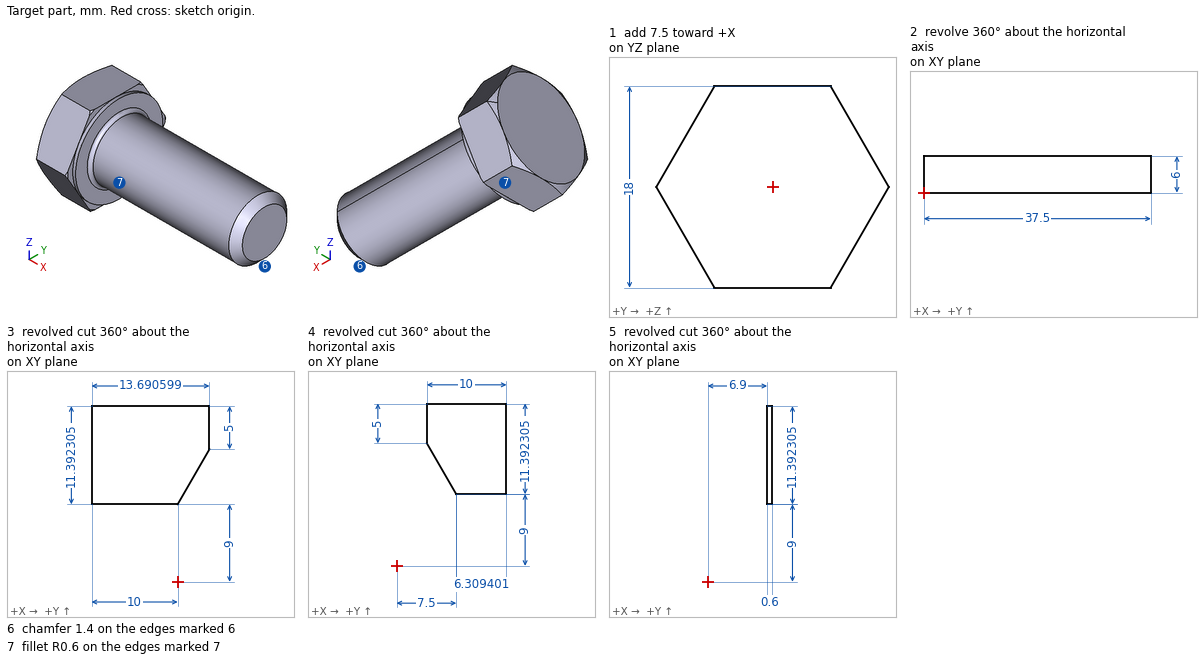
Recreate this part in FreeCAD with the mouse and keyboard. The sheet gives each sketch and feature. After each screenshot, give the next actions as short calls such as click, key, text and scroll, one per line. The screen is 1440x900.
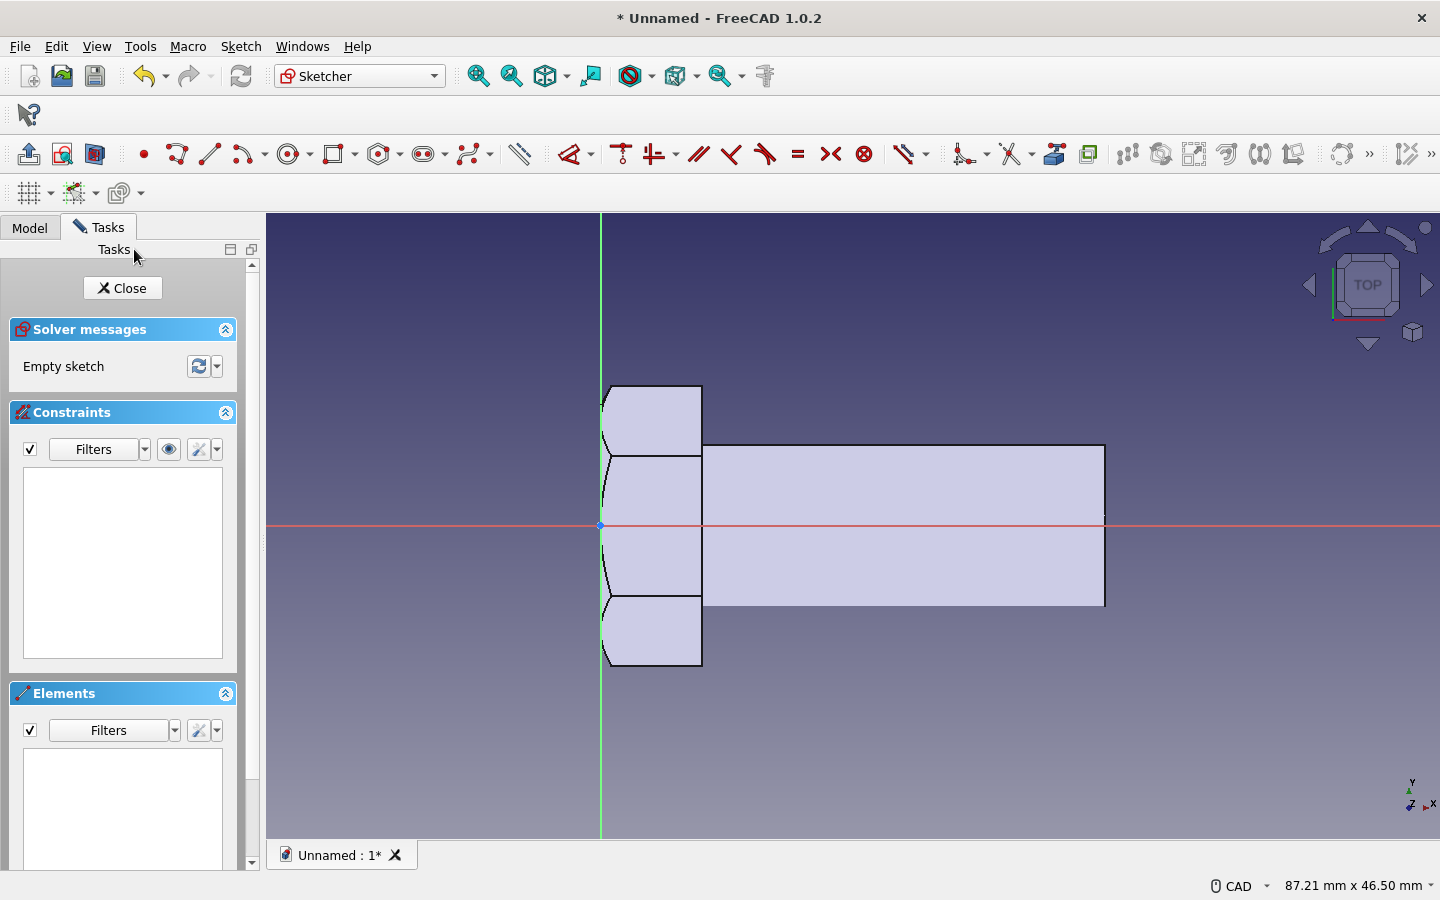
scroll(1195, 811, down, 1)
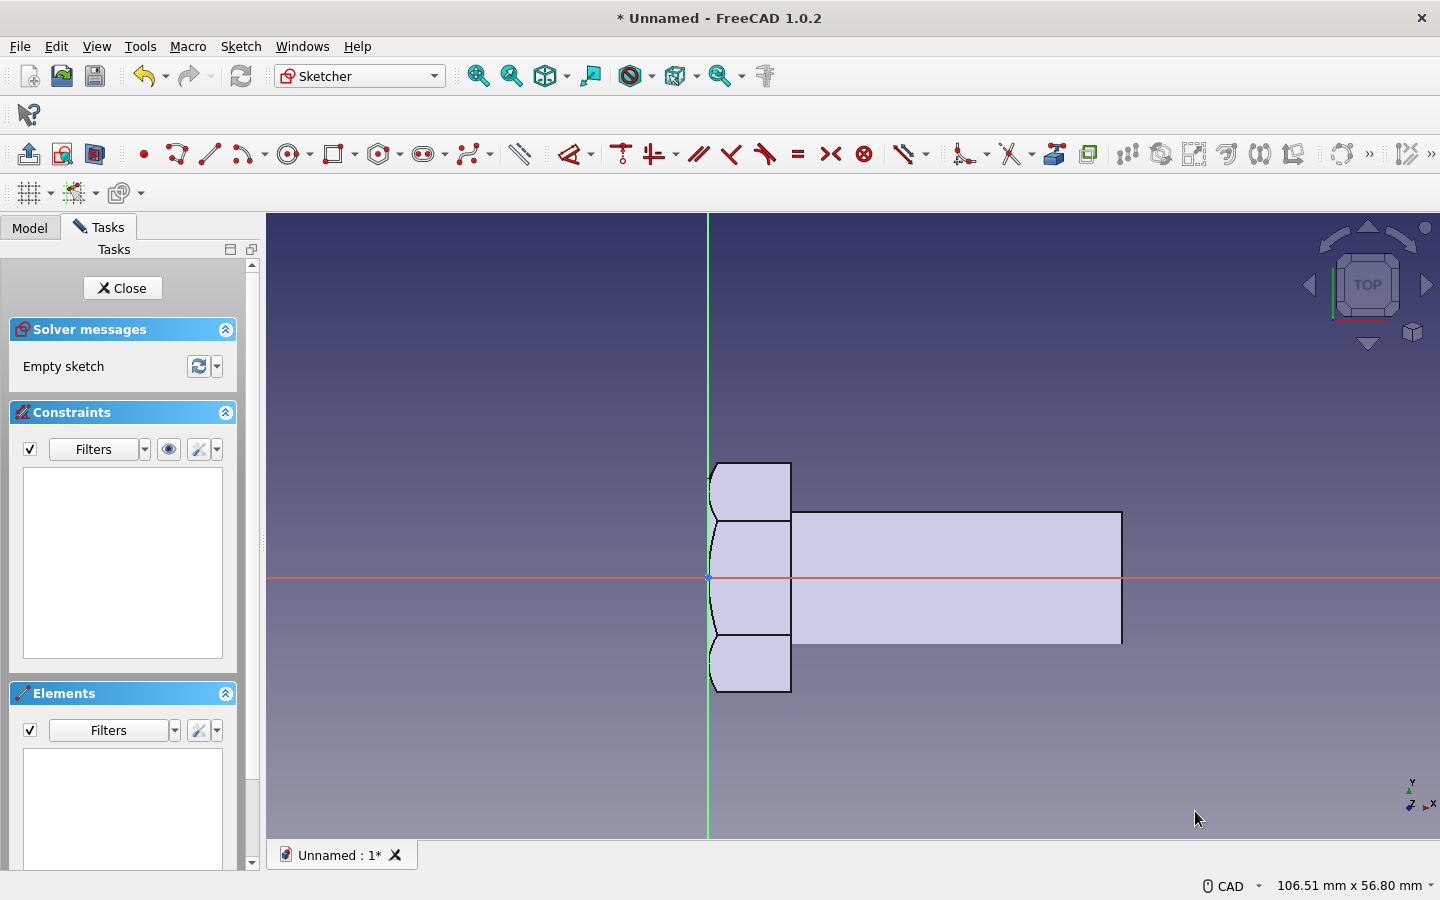
scroll(785, 392, up, 3)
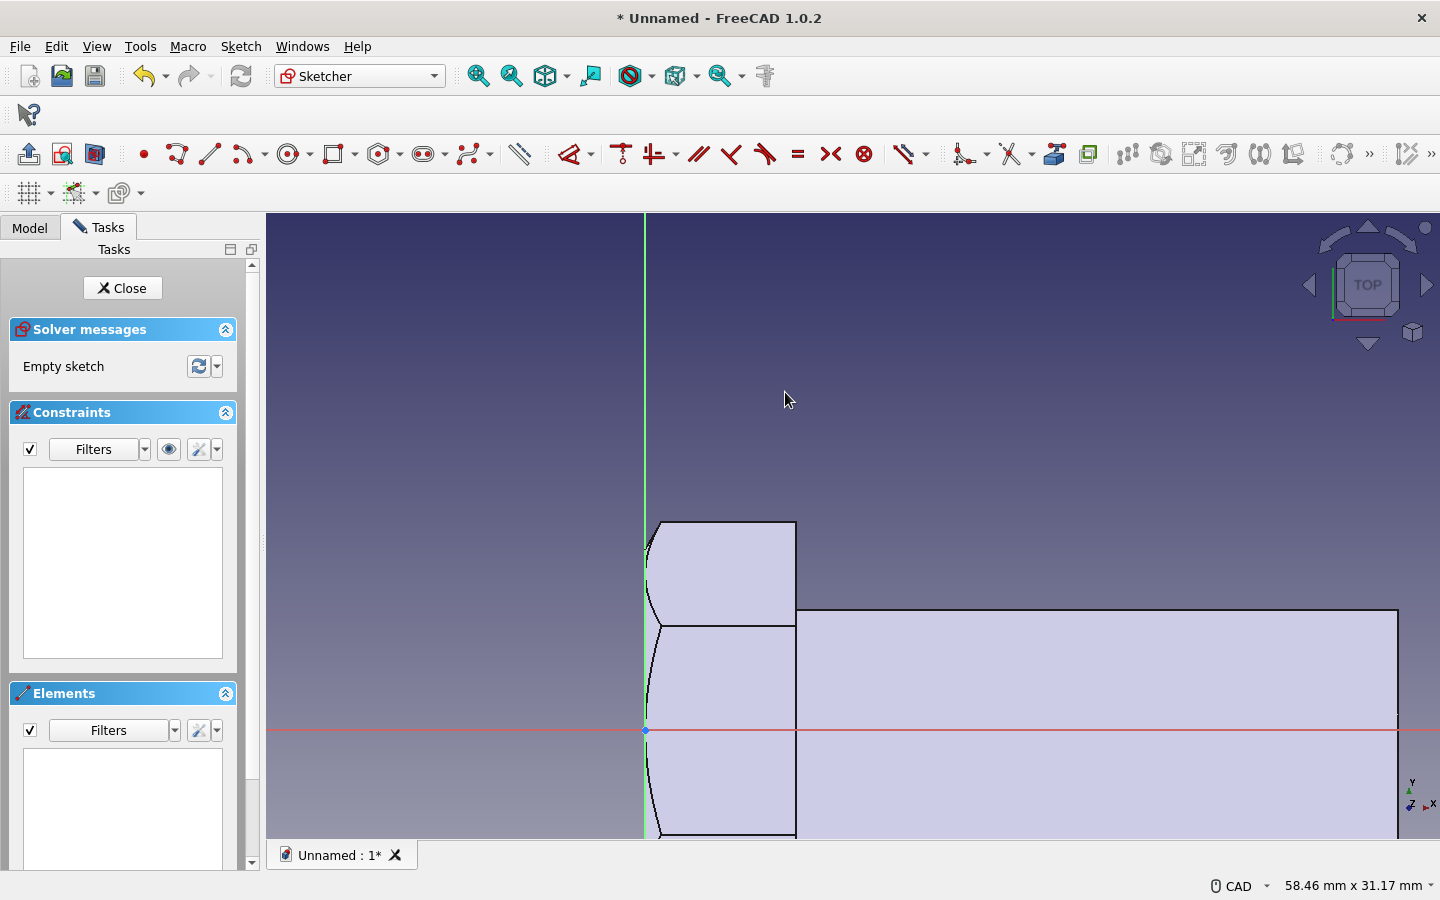
key(g)
key(m)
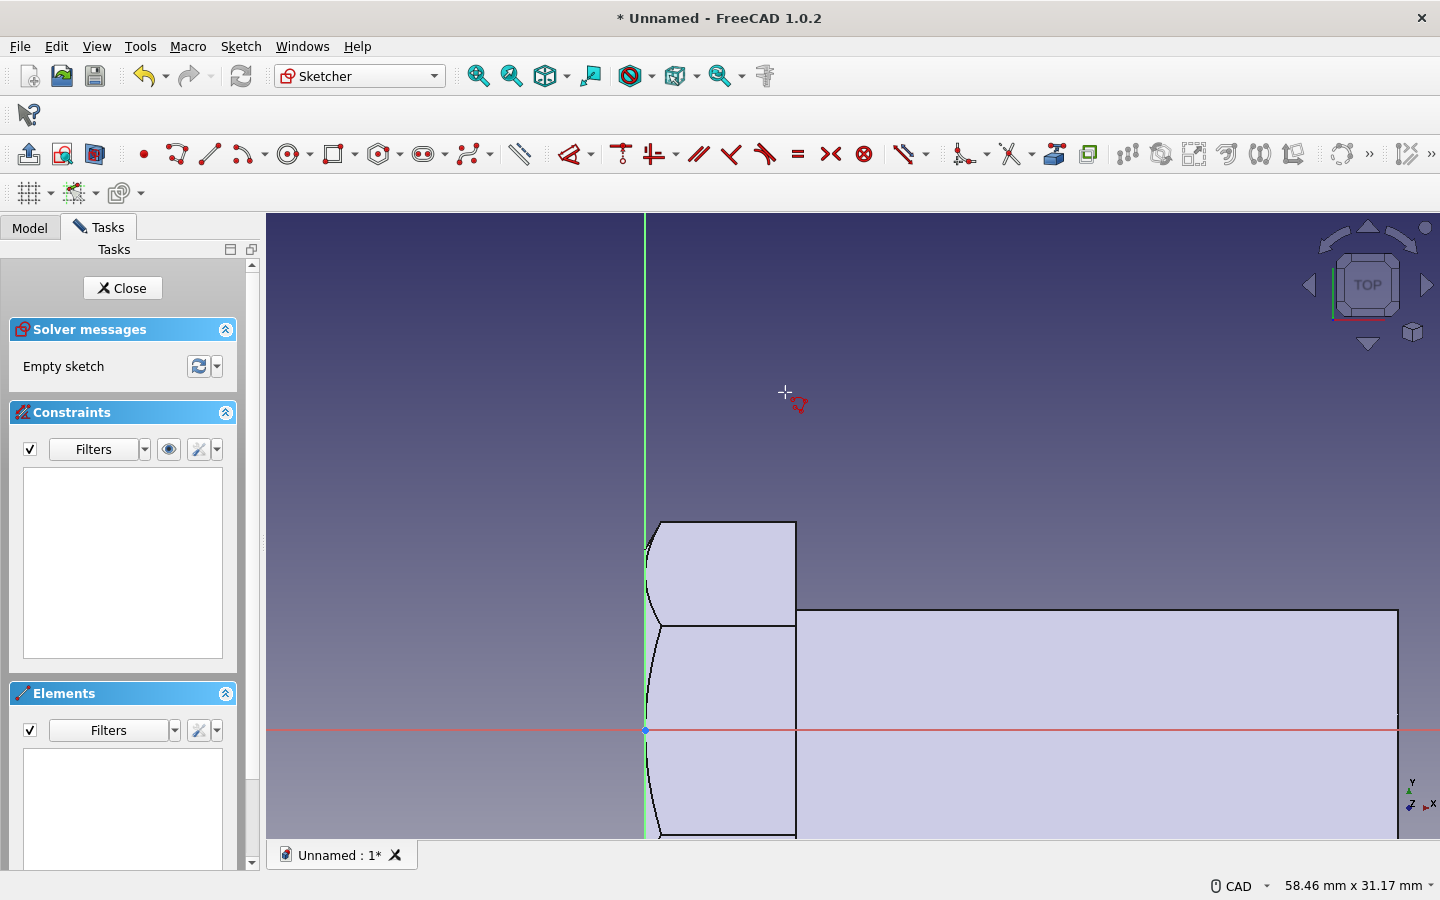
click(796, 550)
click(923, 550)
click(923, 321)
click(722, 321)
click(722, 421)
click(796, 551)
key(Escape)
key(Escape)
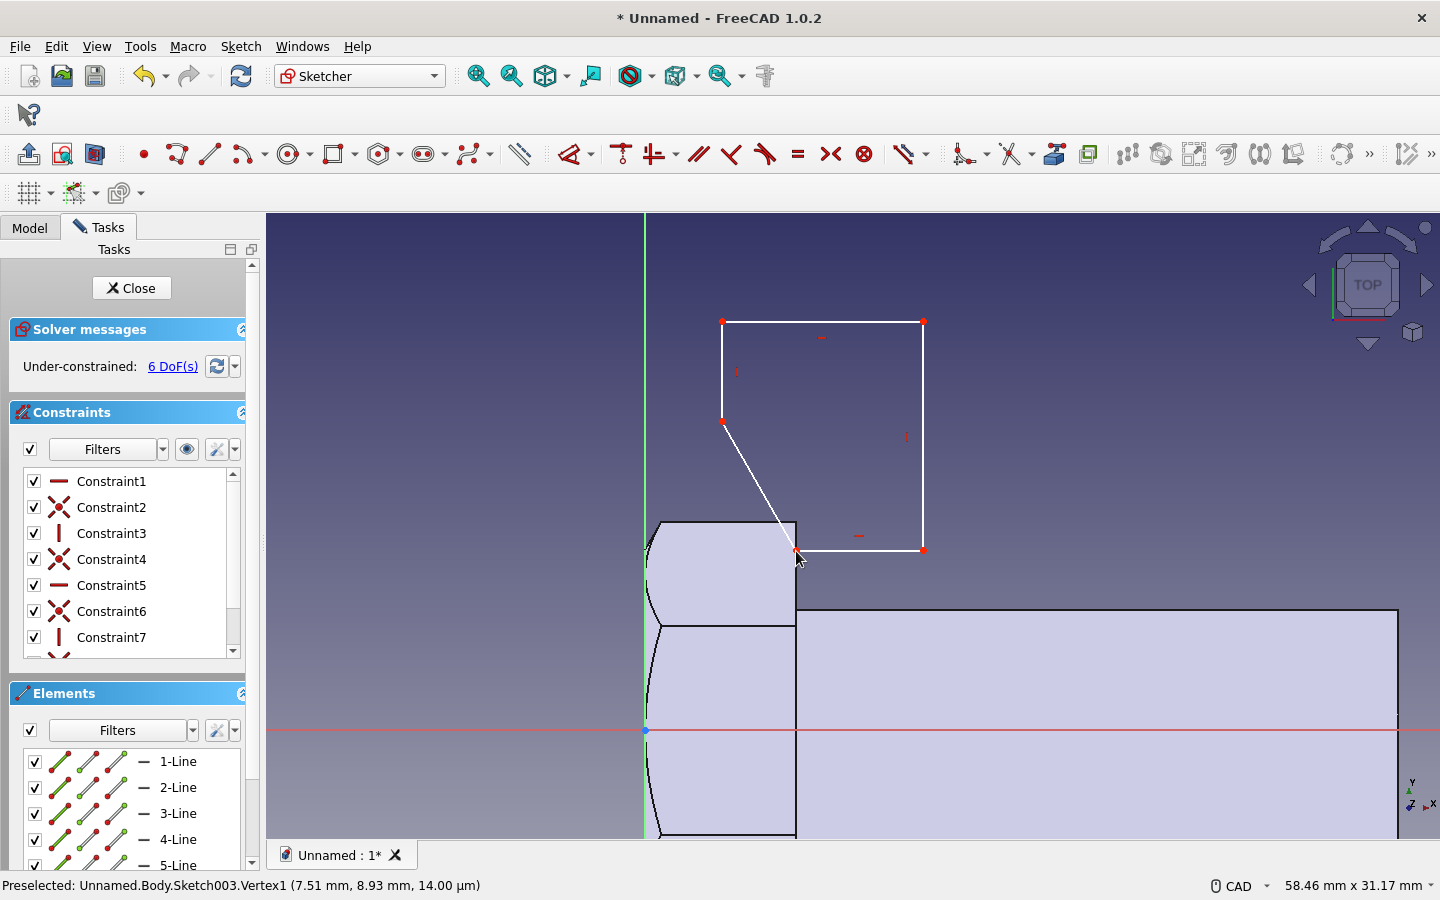
key(d)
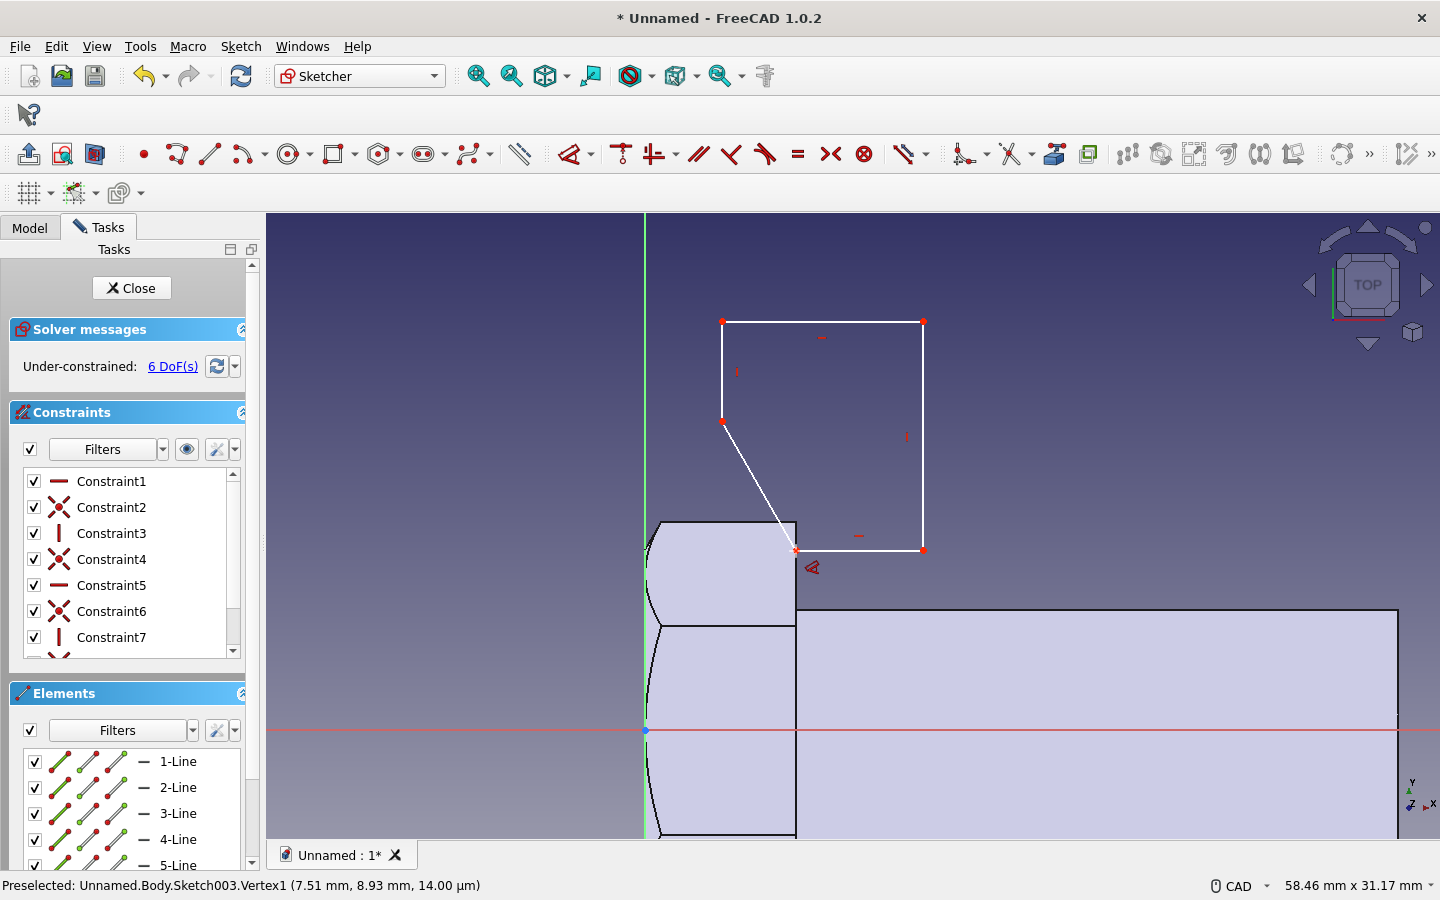
click(722, 352)
click(688, 372)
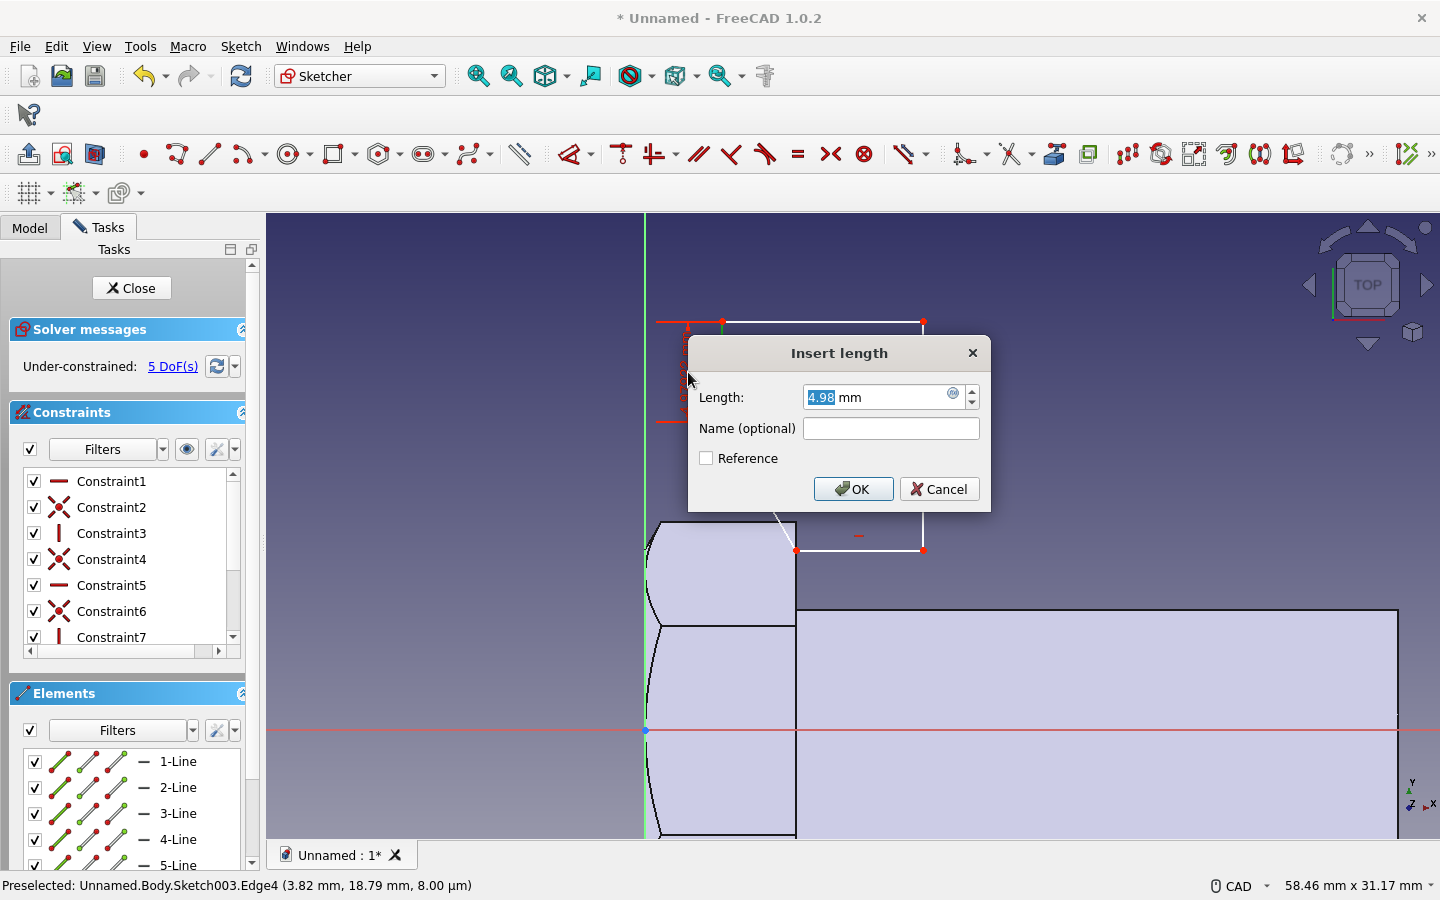
text(5)
key(Return)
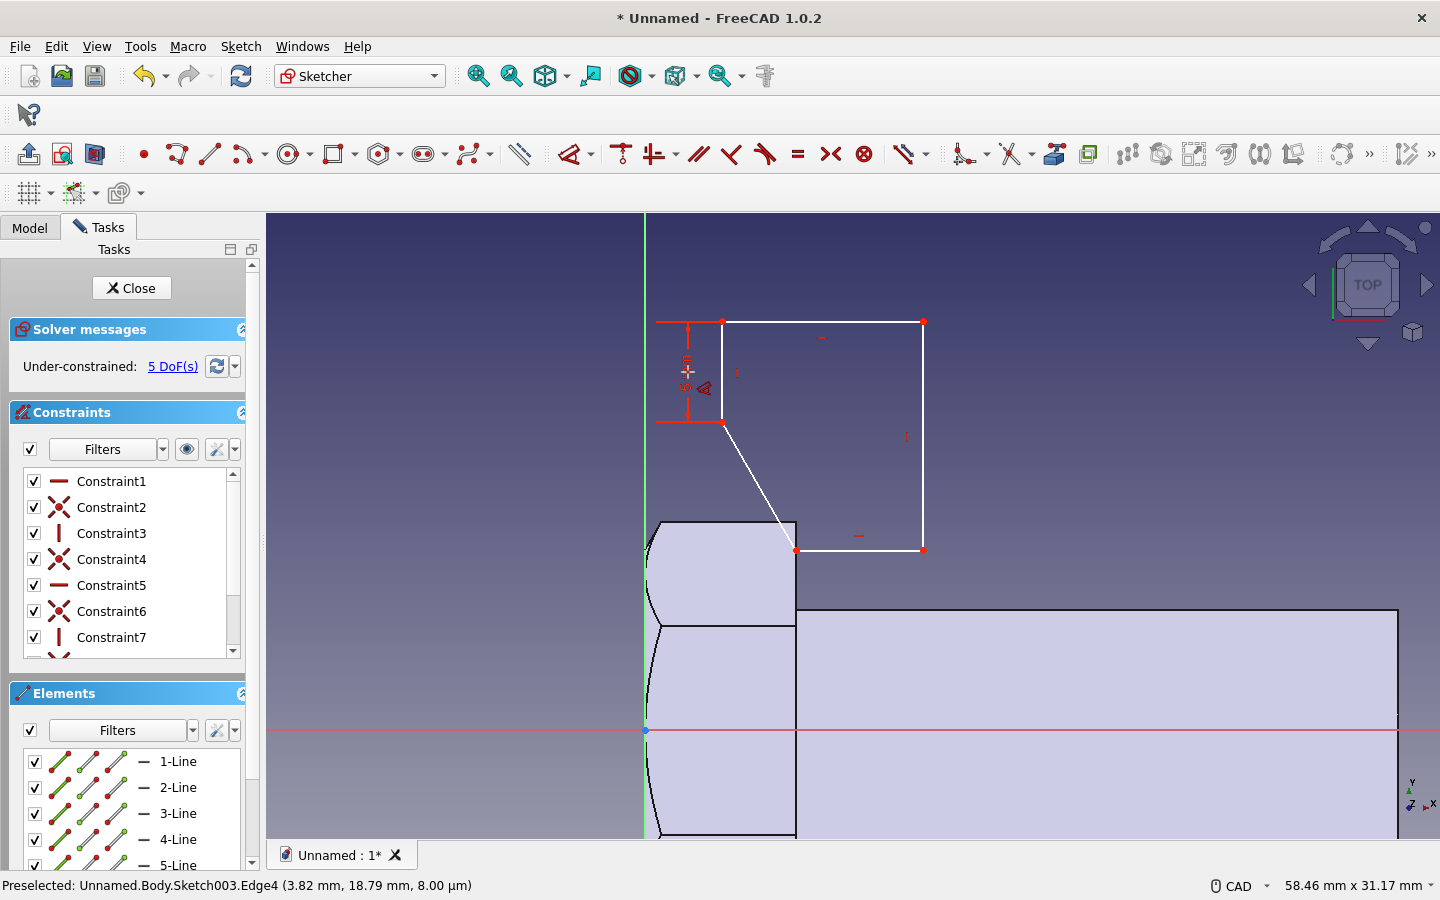
click(863, 322)
click(822, 288)